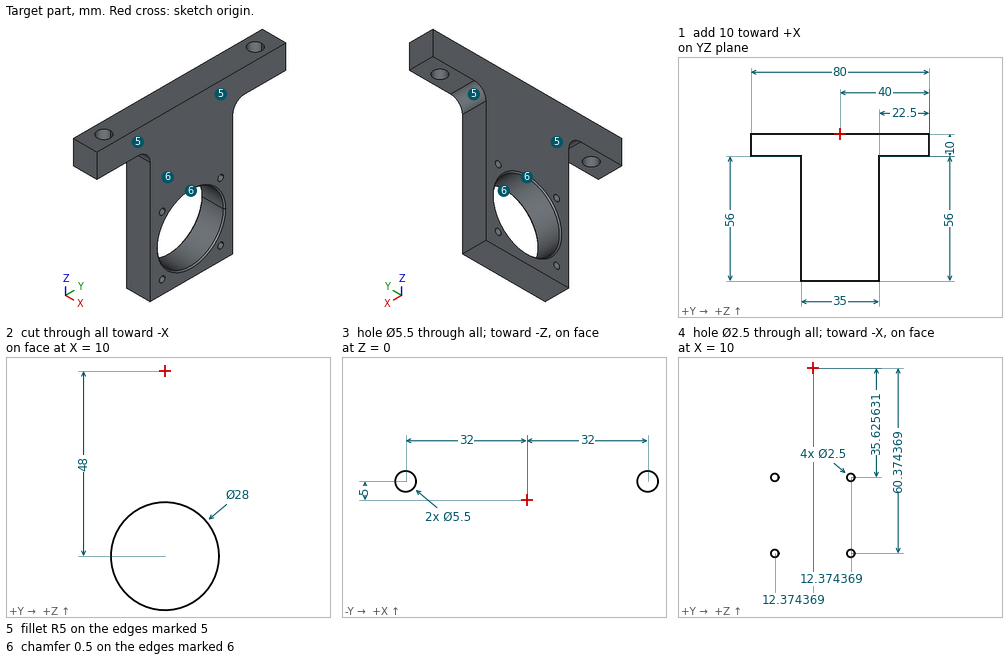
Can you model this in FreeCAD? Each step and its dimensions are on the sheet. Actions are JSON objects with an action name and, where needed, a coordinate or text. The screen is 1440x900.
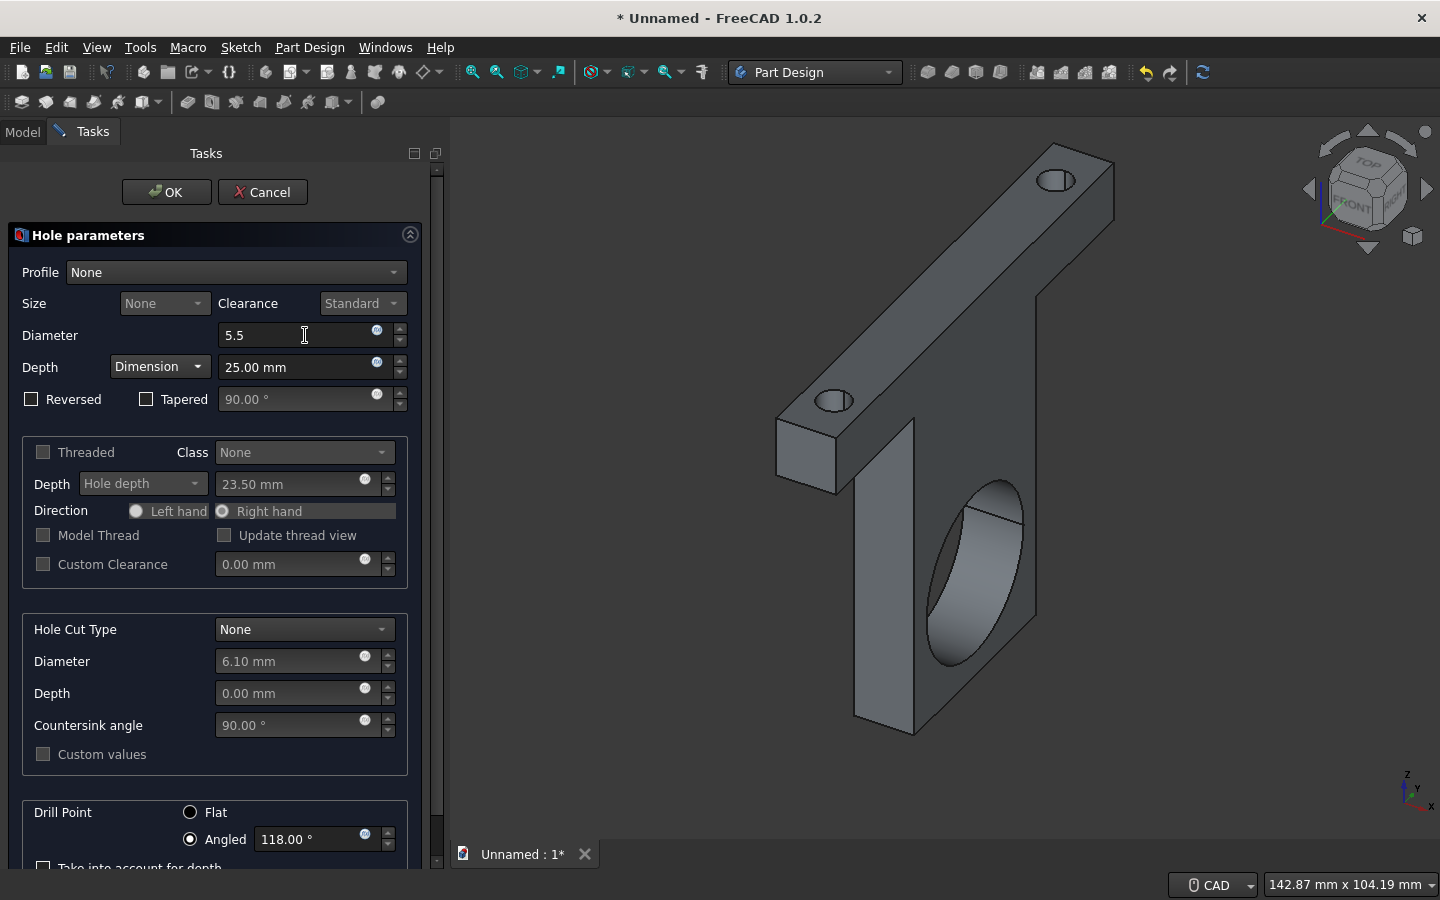
{"action": "left_click", "coordinate": [161, 366]}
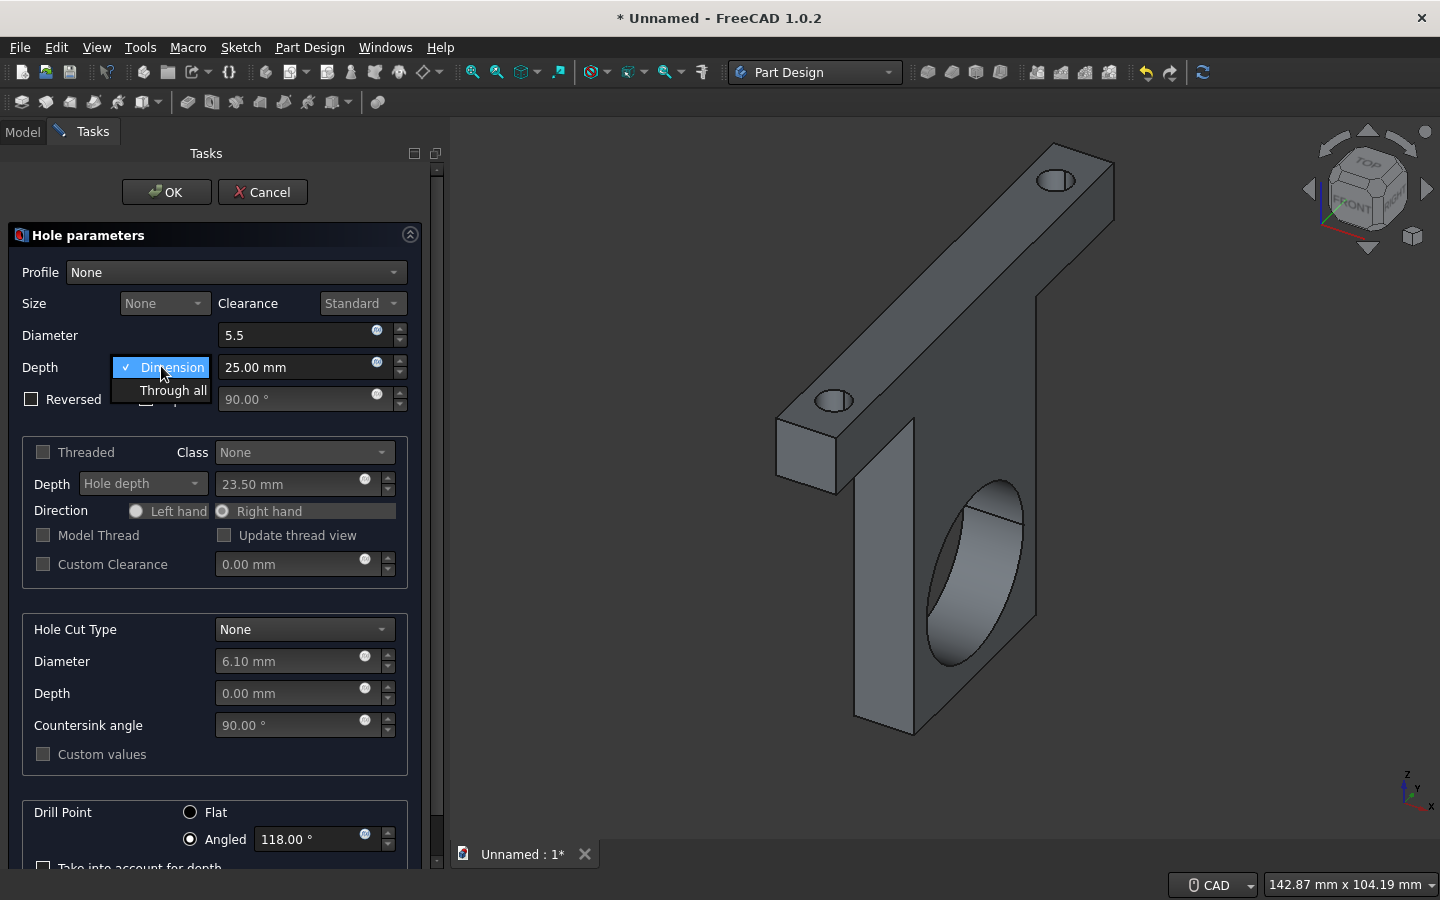
{"action": "left_click", "coordinate": [160, 390]}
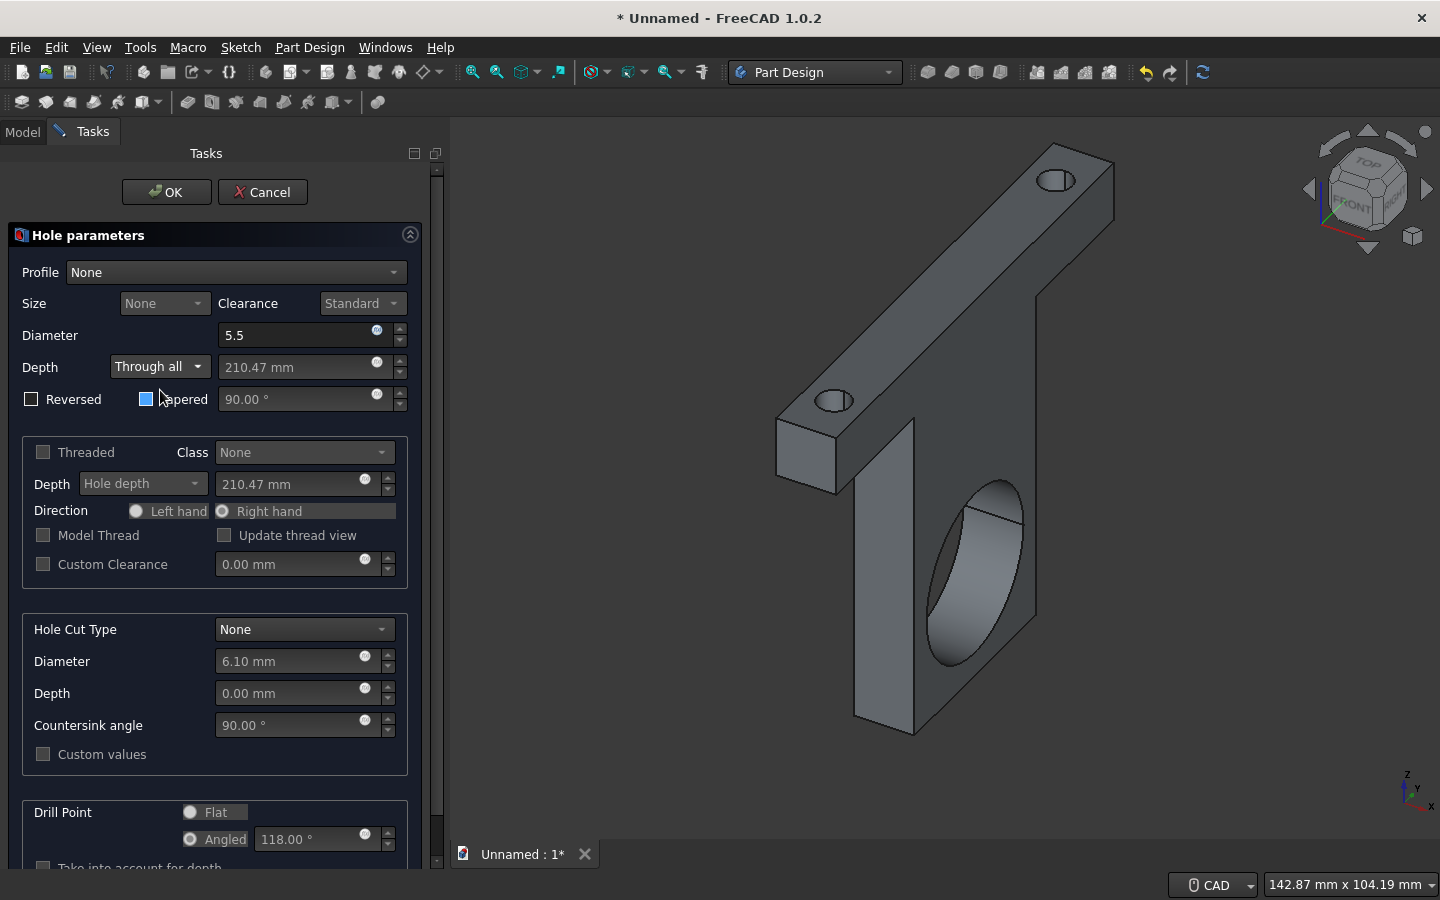
{"action": "left_click", "coordinate": [167, 192]}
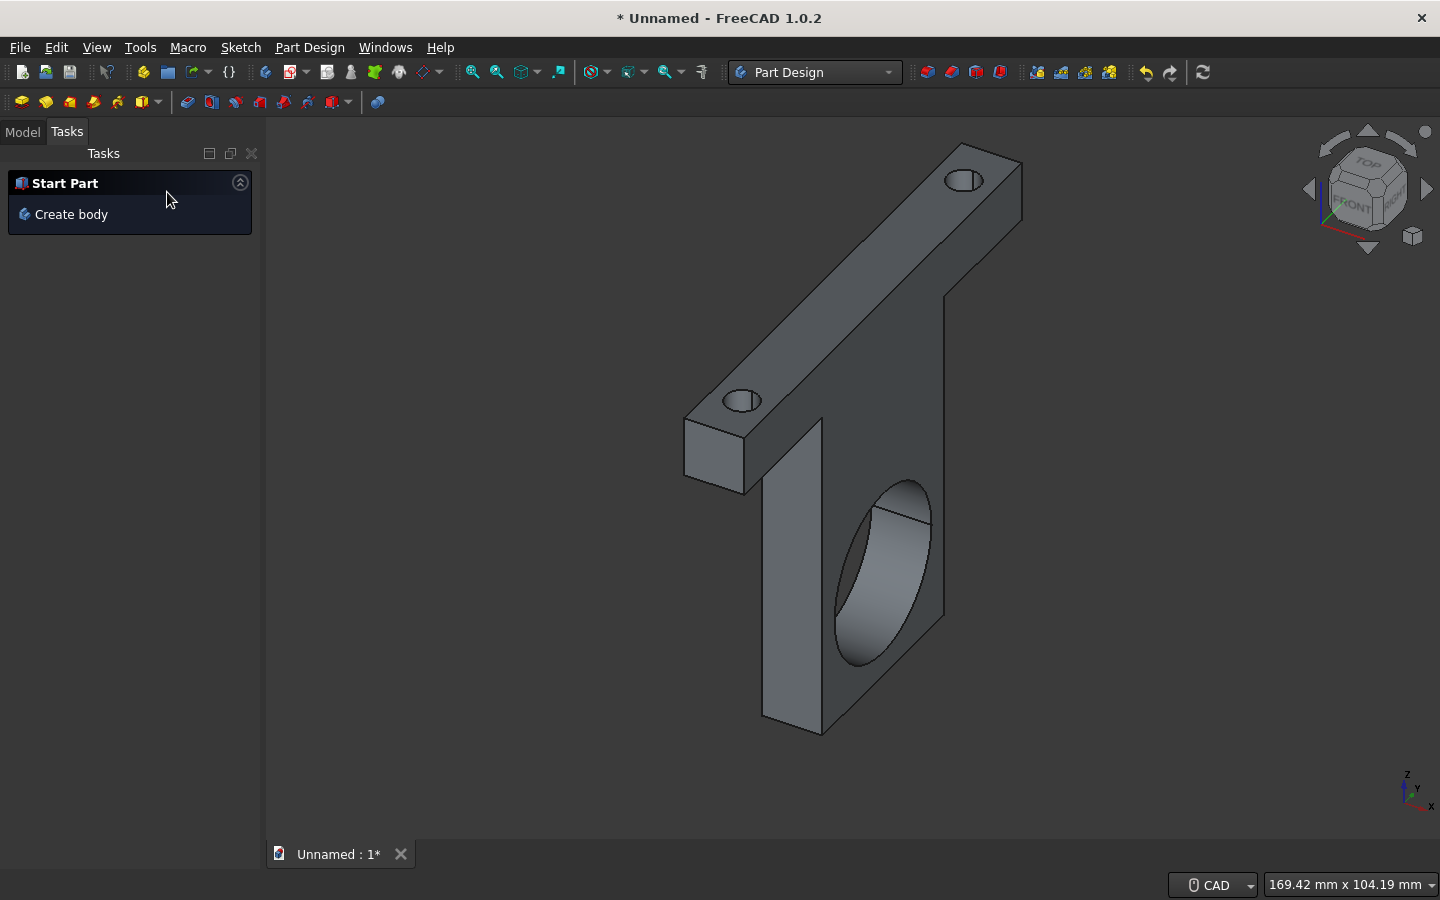
{"action": "left_click", "coordinate": [883, 380]}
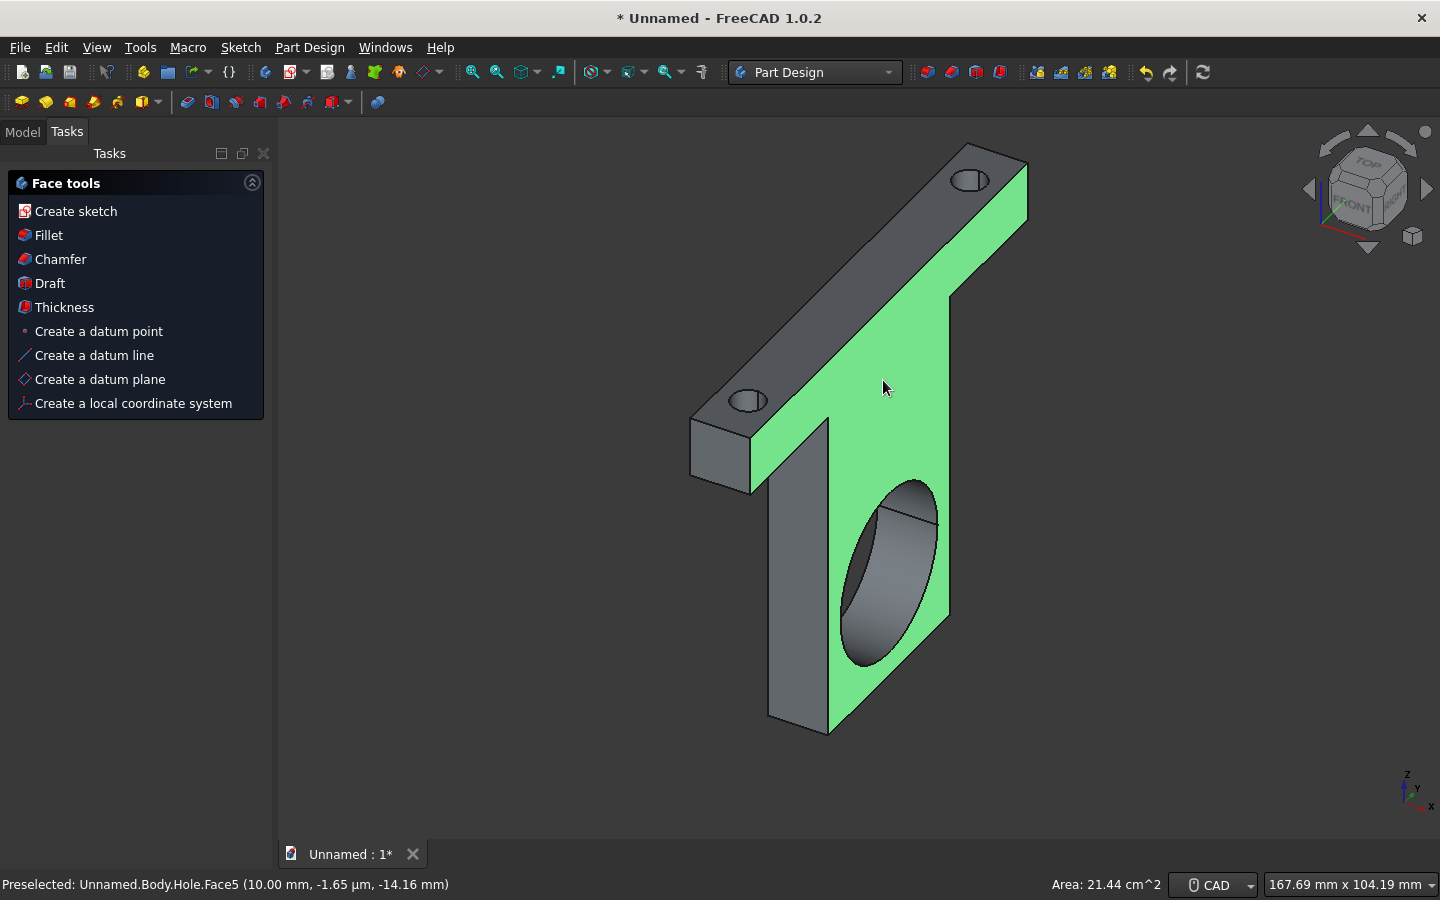
{"action": "left_click", "coordinate": [290, 72]}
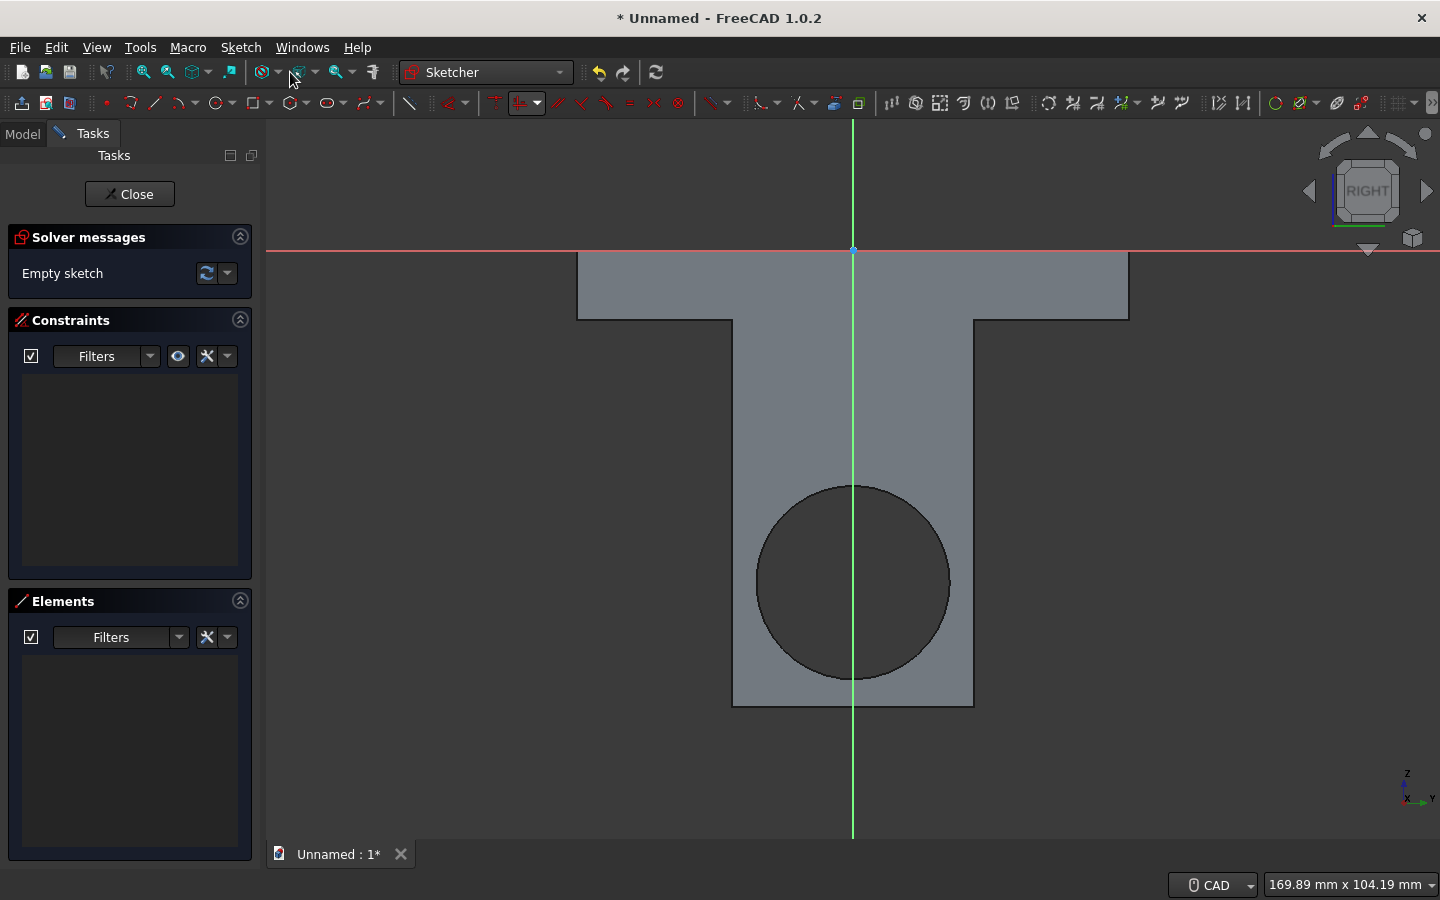
{"action": "left_click", "coordinate": [216, 104]}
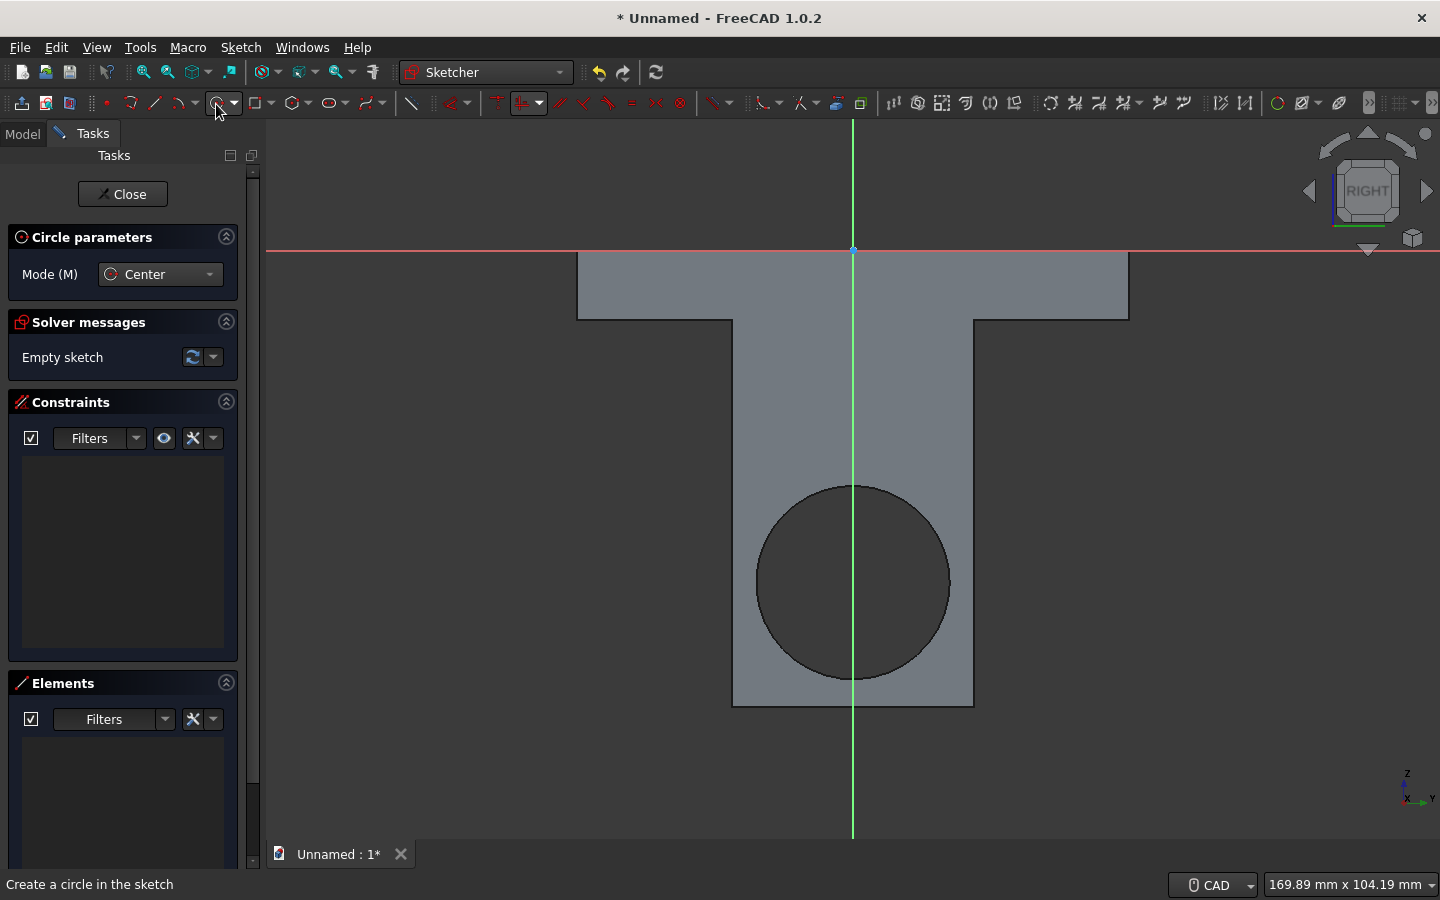
{"action": "scroll", "coordinate": [939, 497], "scroll_direction": "up", "scroll_amount": 5}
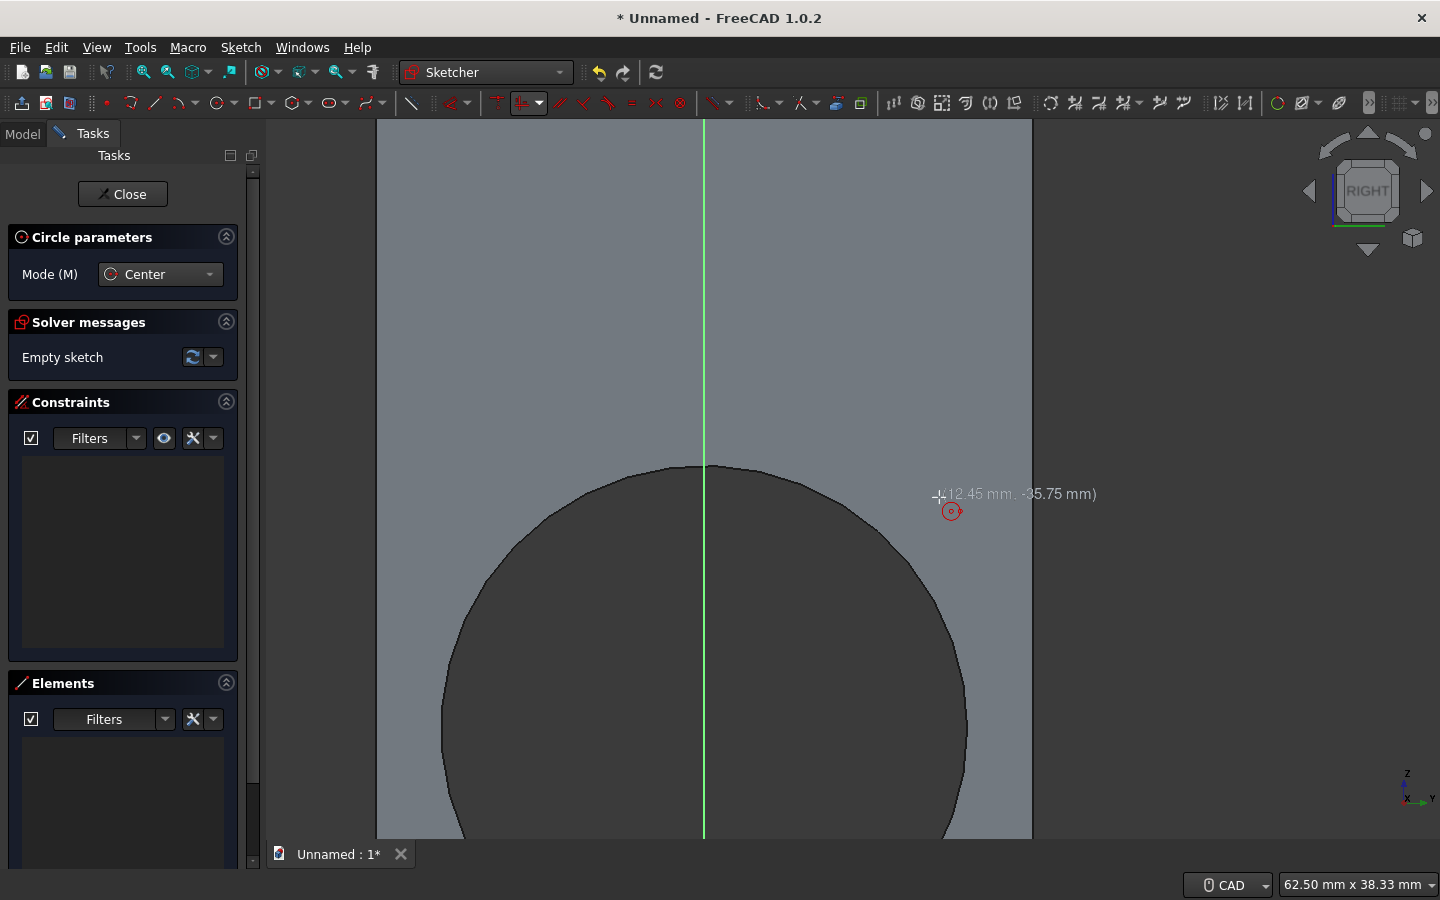
{"action": "left_click", "coordinate": [937, 496]}
{"action": "mouse_move", "coordinate": [953, 480]}